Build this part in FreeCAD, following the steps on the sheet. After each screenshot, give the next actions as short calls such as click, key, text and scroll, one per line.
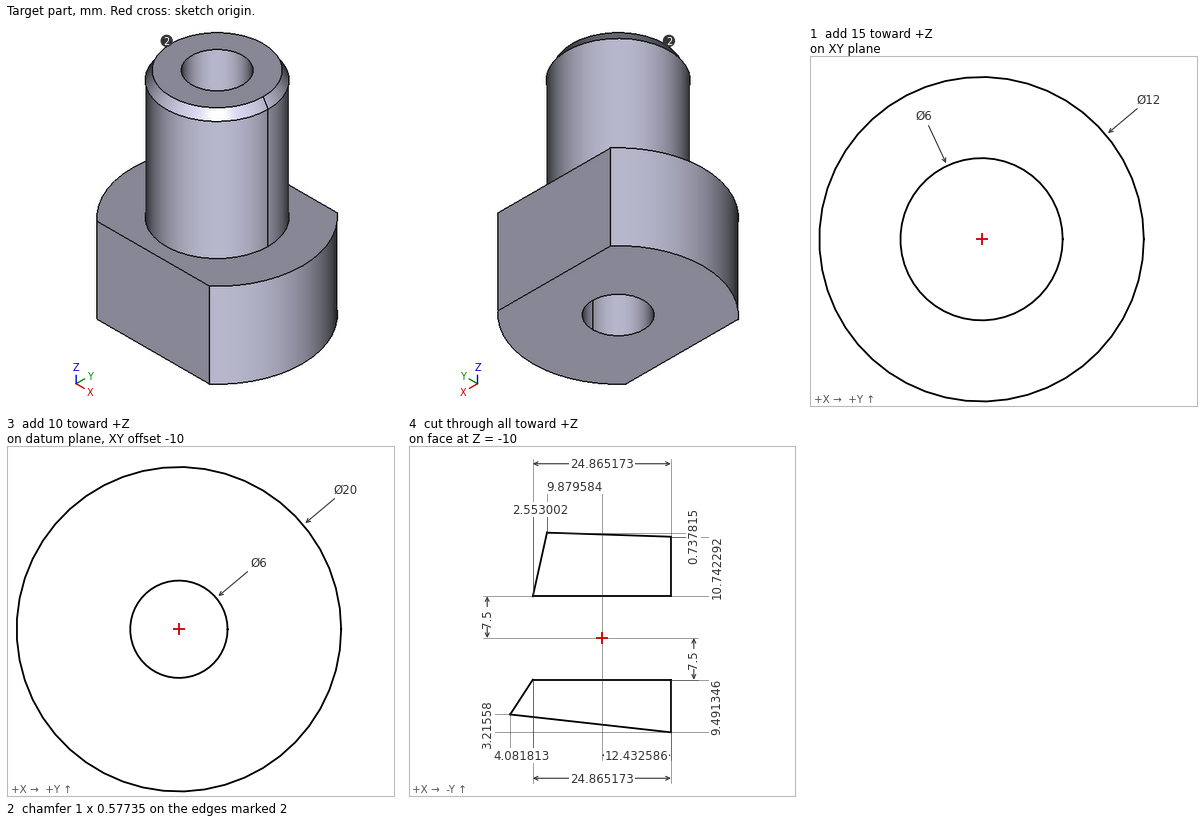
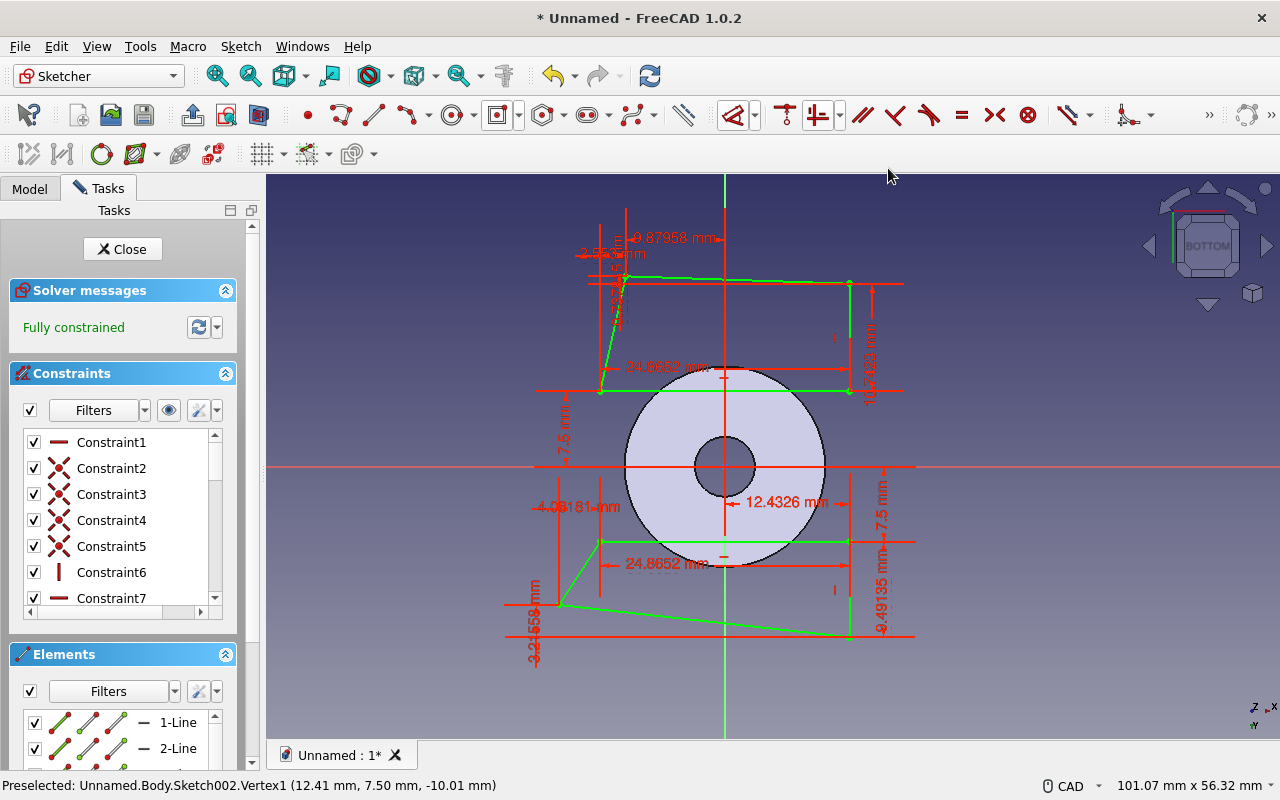
click(123, 249)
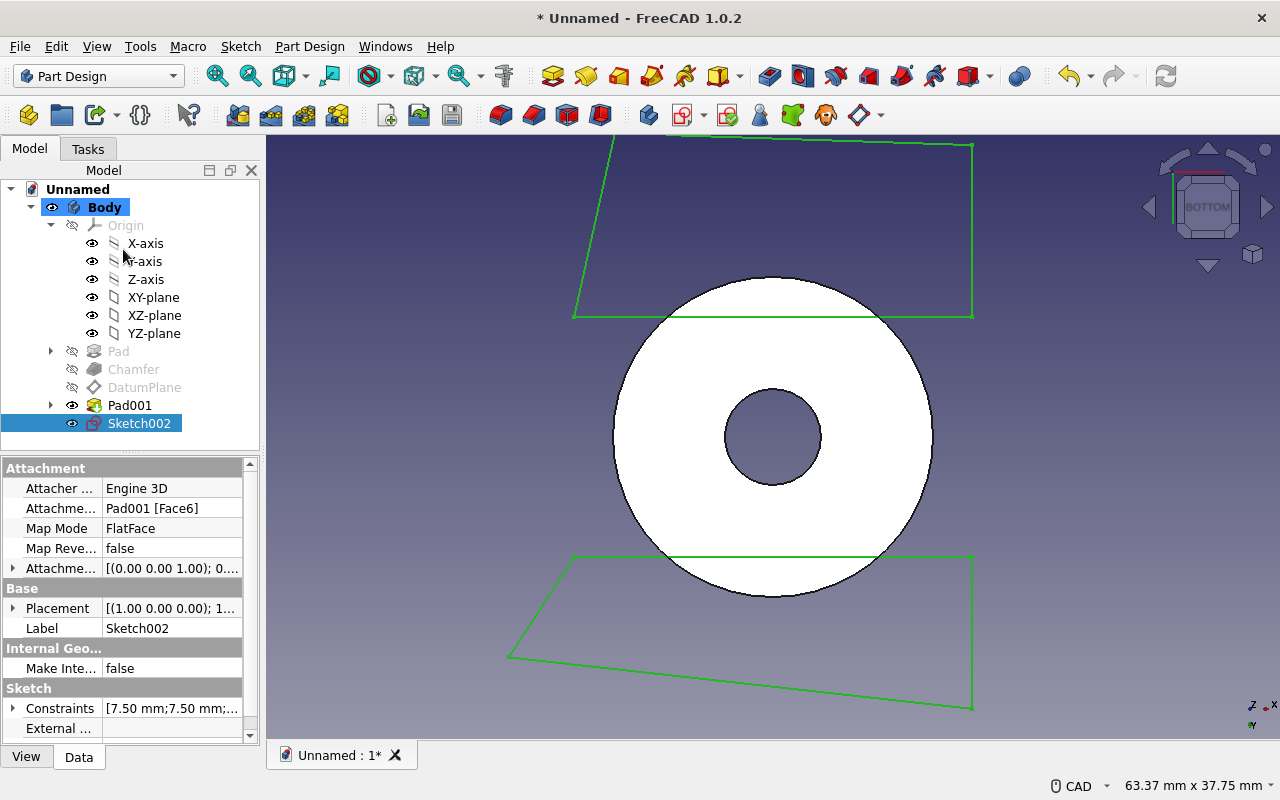
click(770, 76)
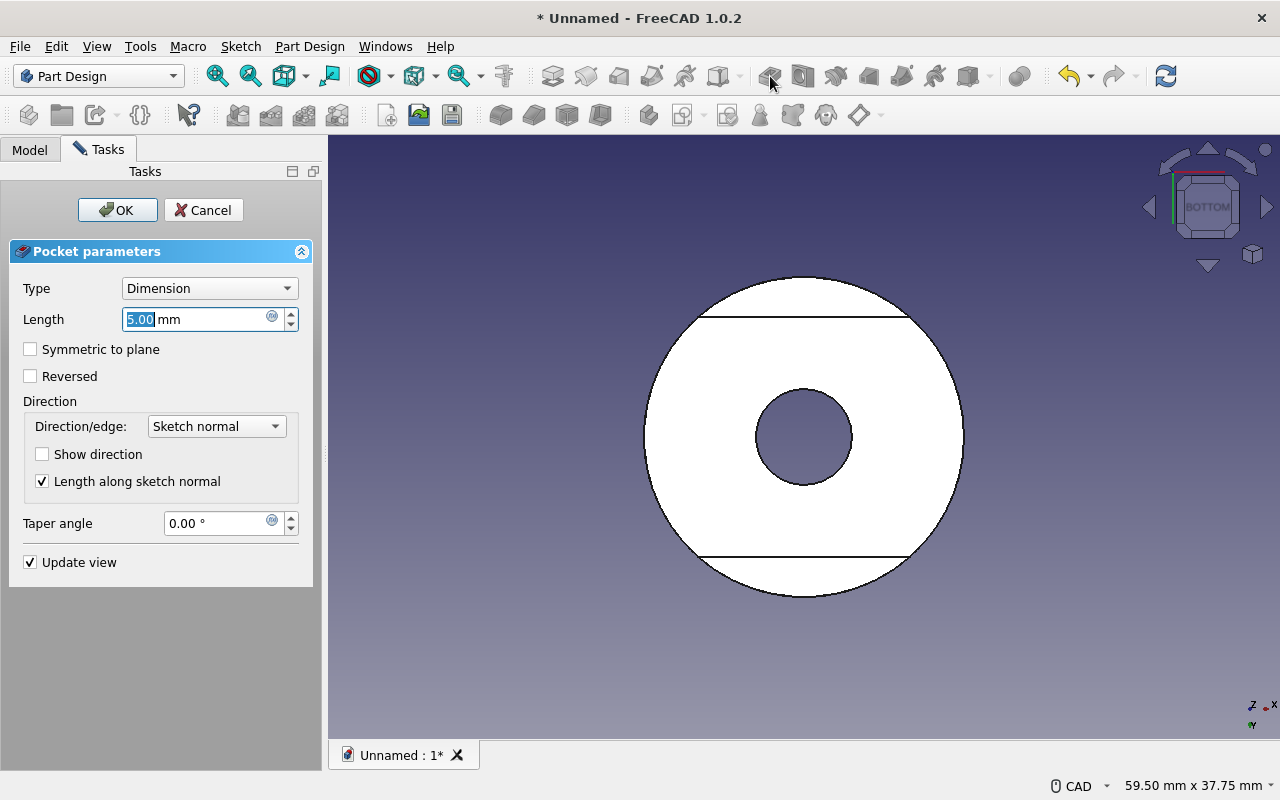
click(210, 288)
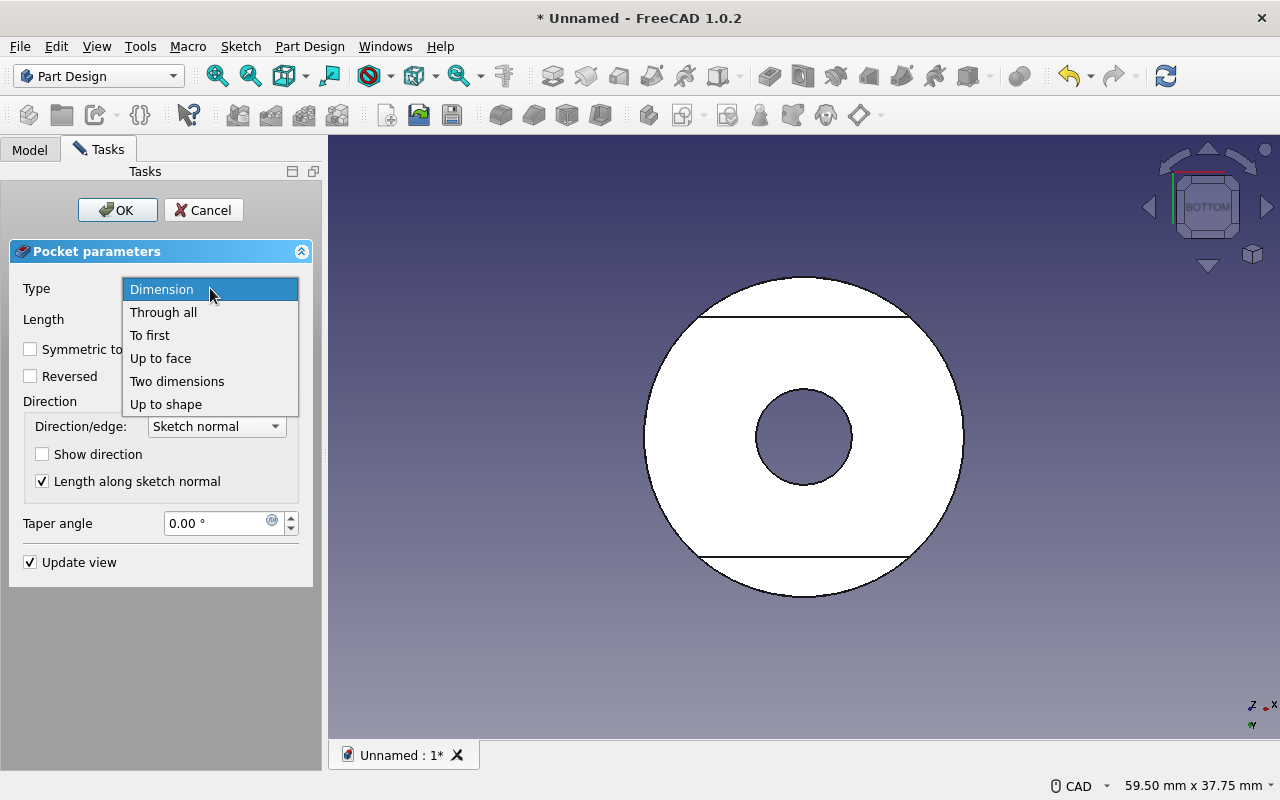
click(208, 312)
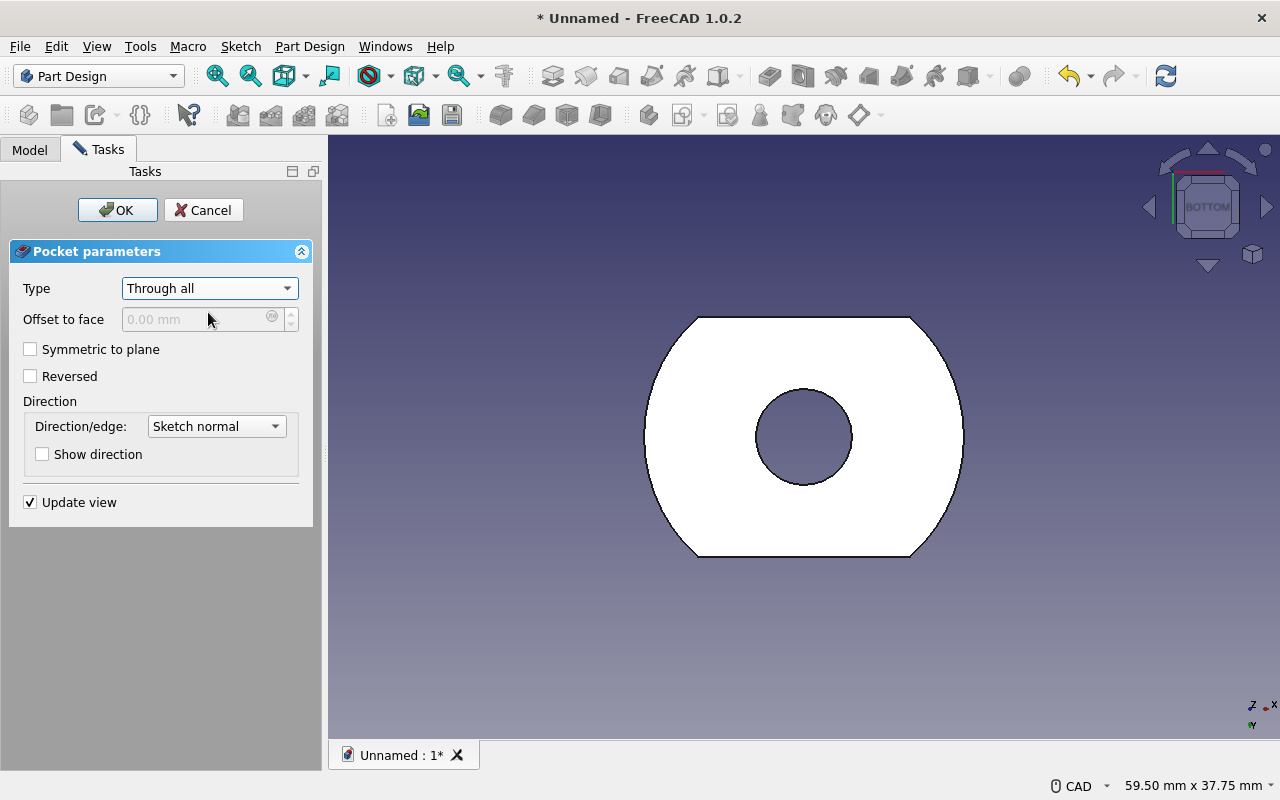
click(118, 210)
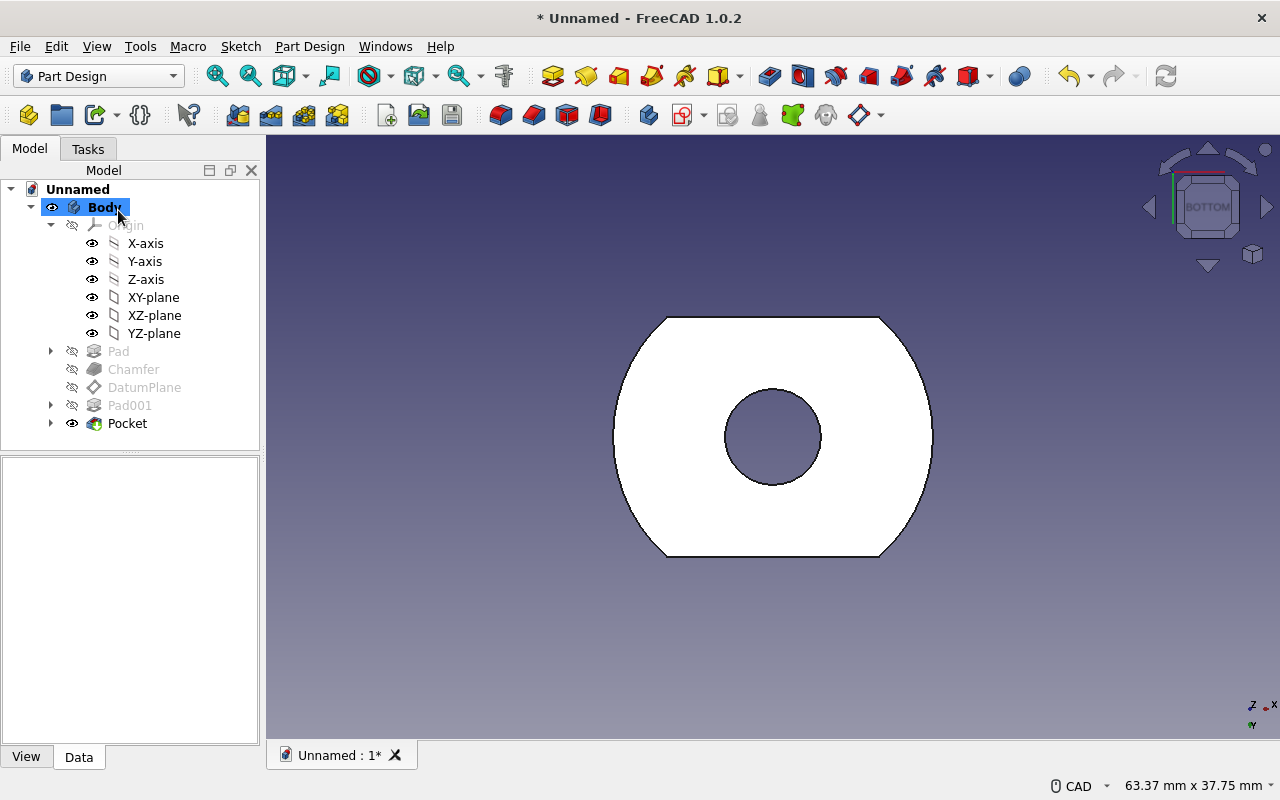
key(0)